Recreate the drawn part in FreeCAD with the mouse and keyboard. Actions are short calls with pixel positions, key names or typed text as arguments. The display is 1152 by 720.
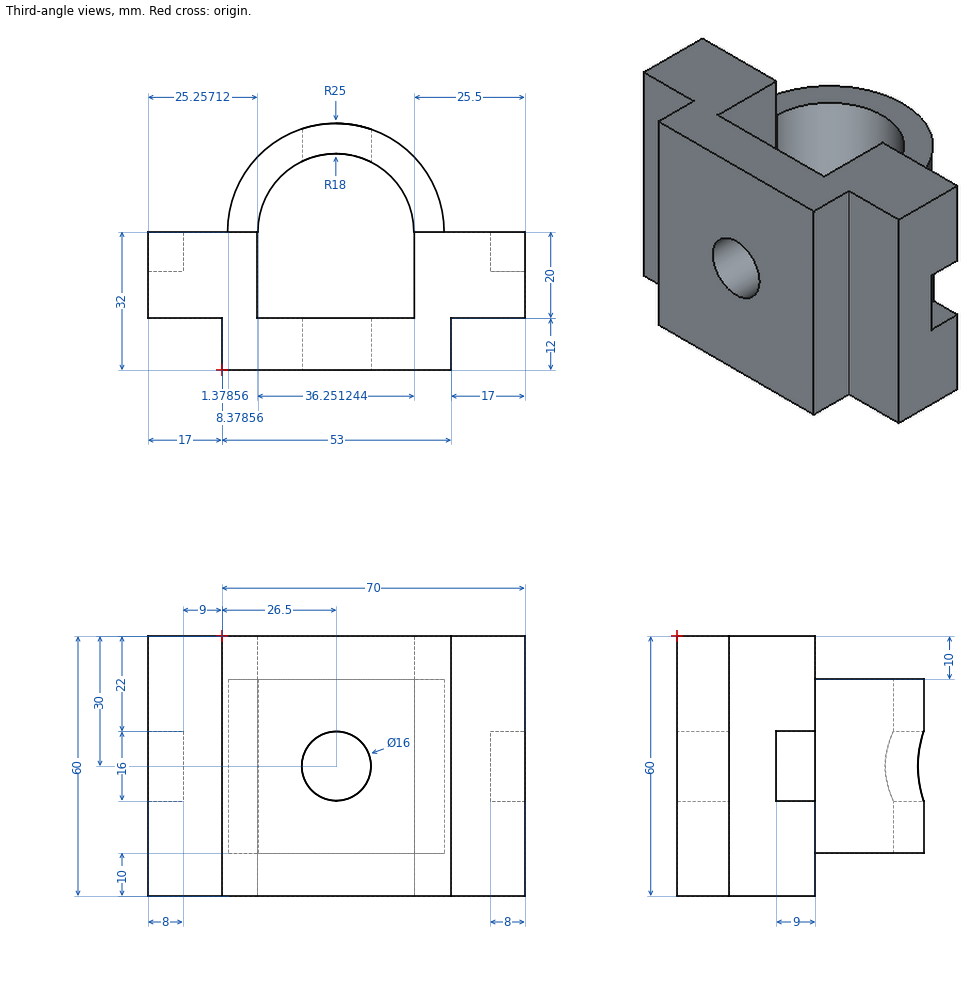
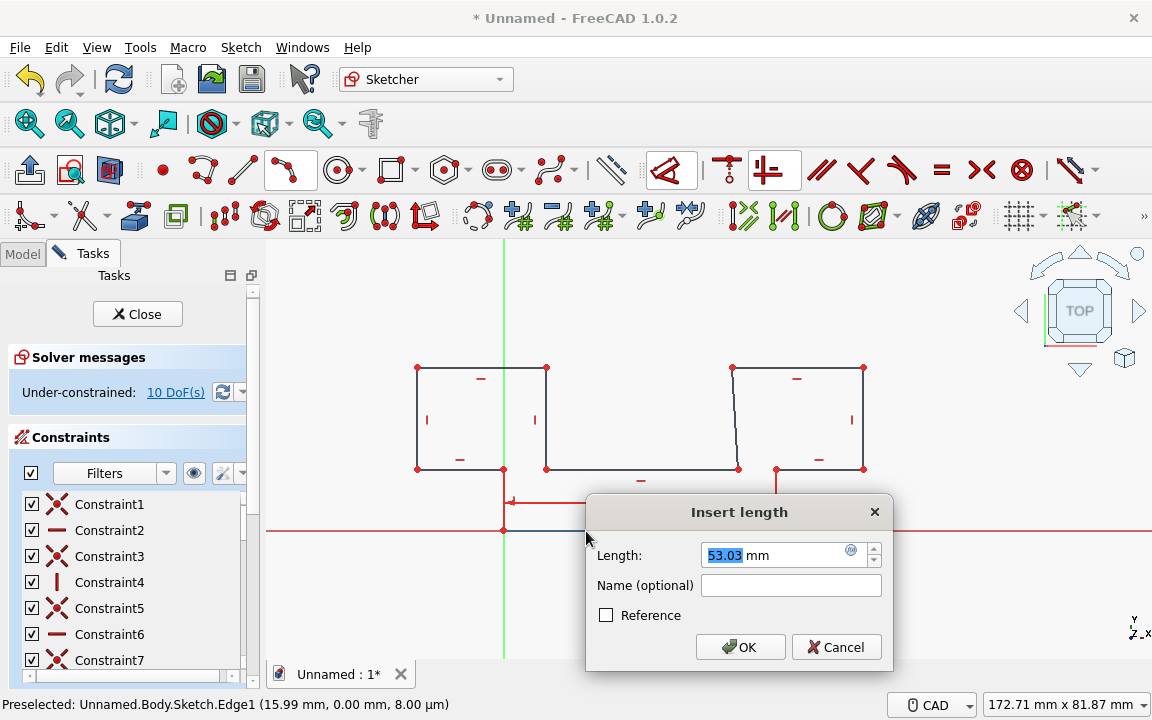
text(53)
key(Return)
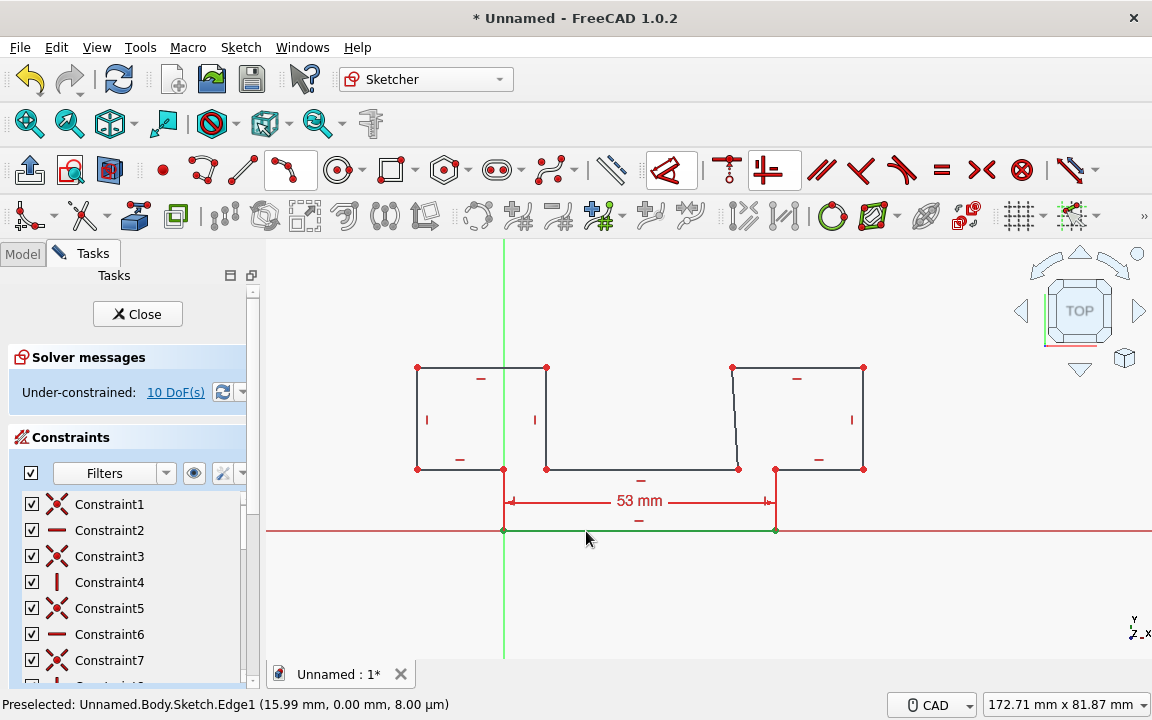
click(776, 513)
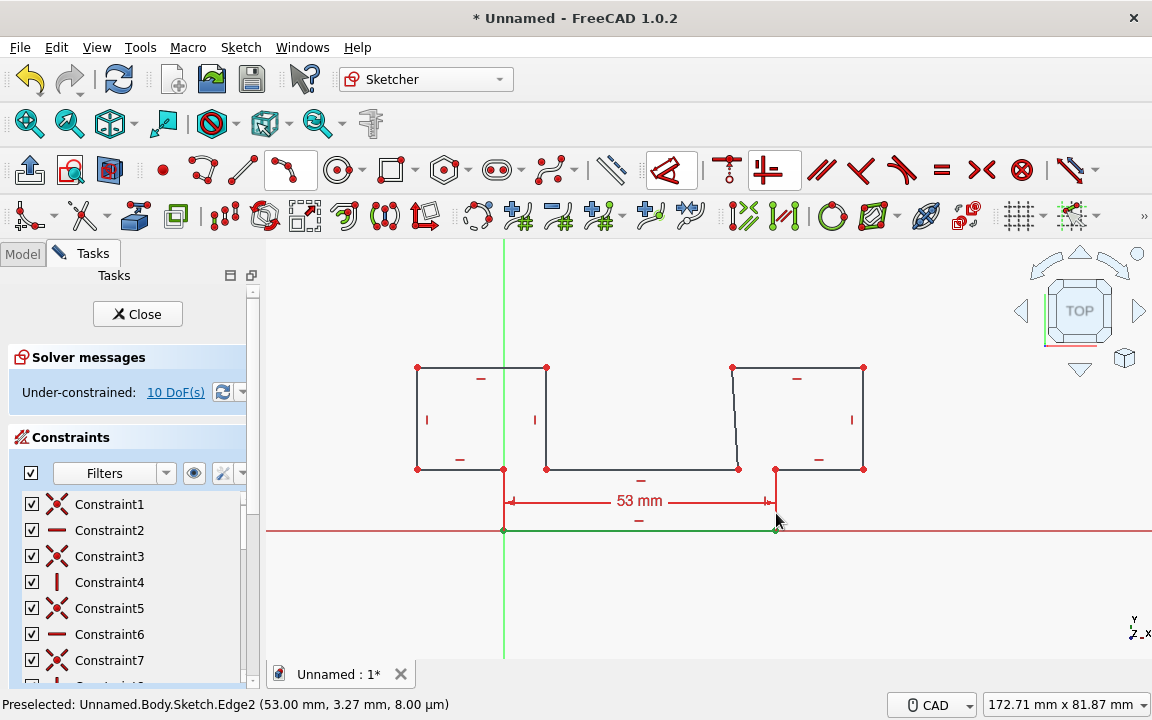
key(i)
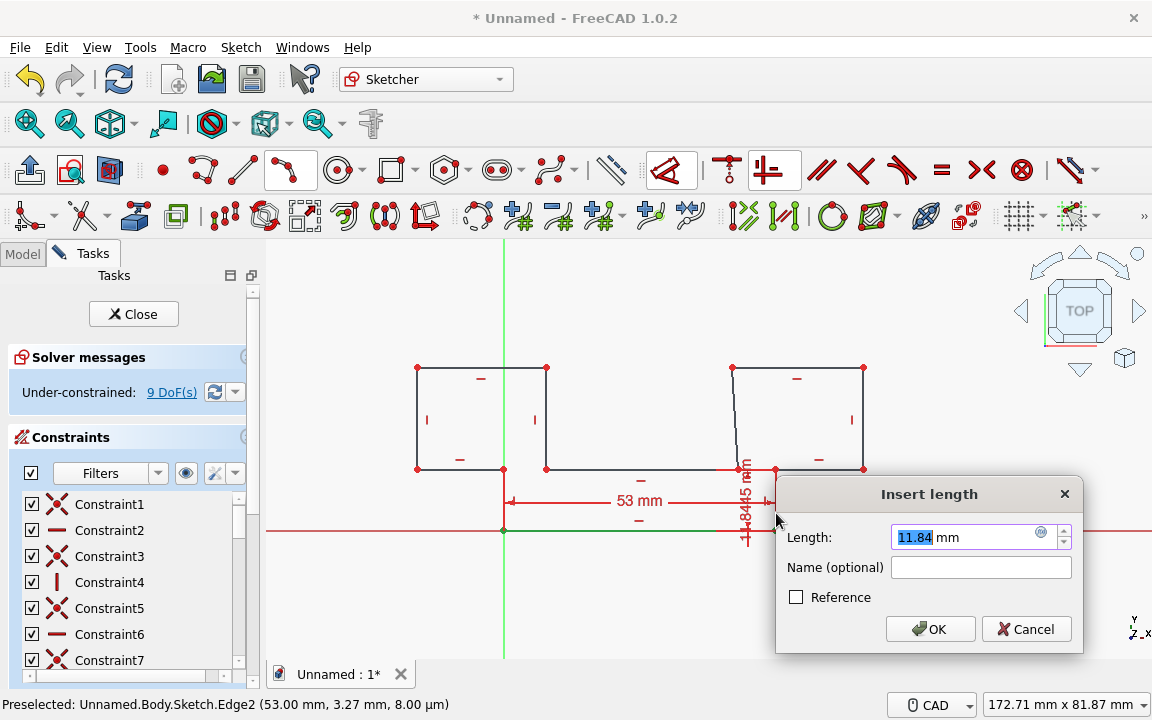
text(12)
key(Return)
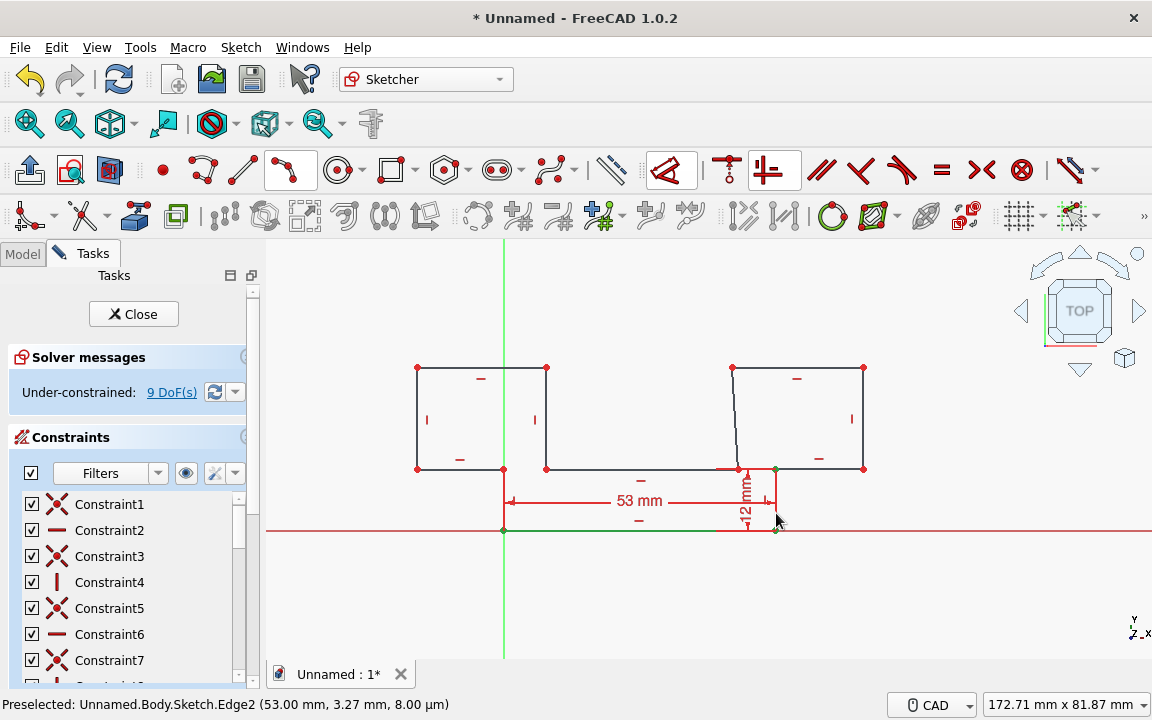
click(802, 469)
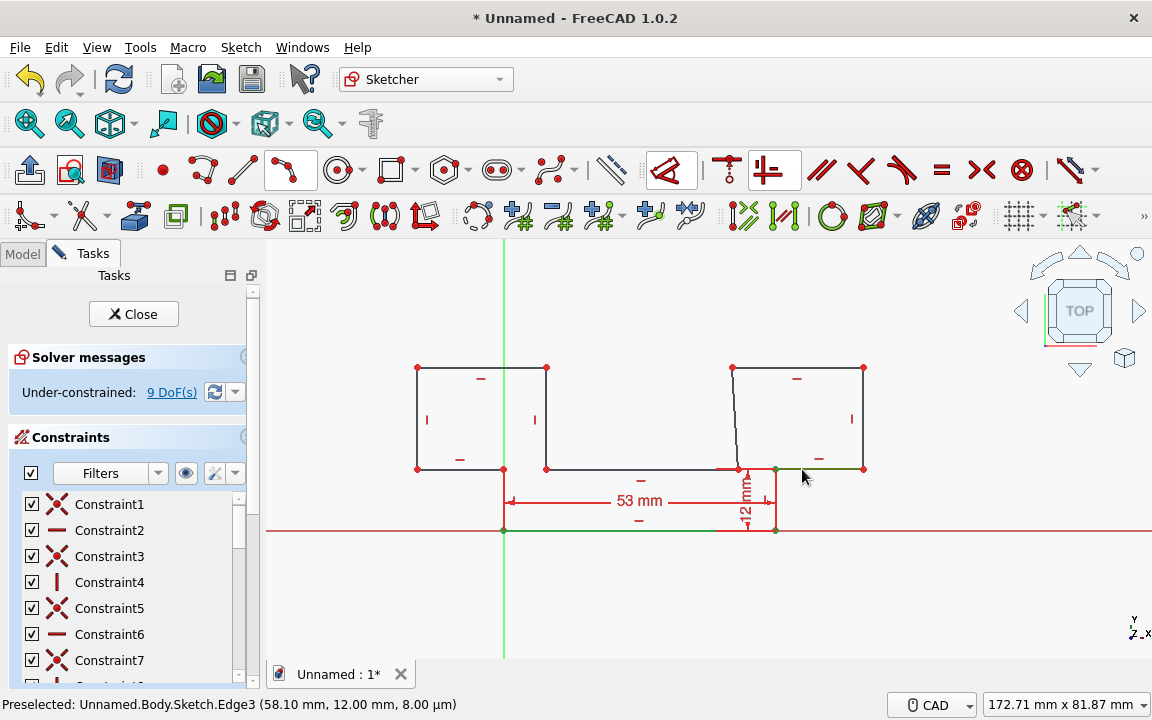
key(l)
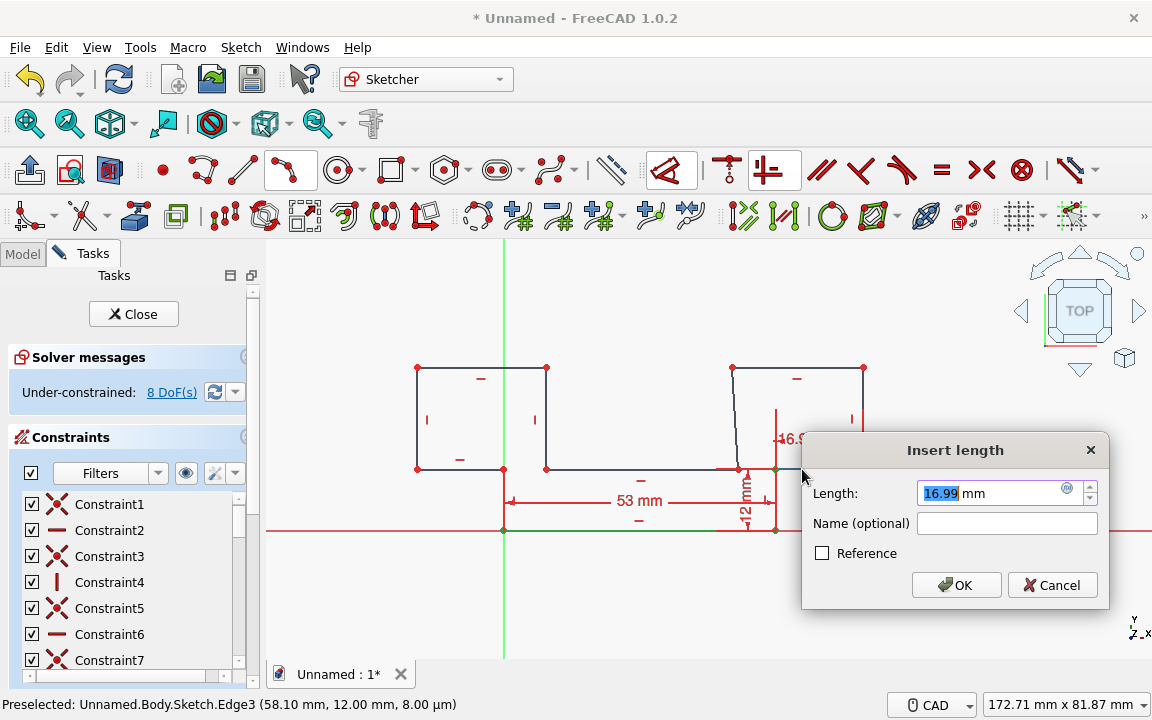
text(17)
key(Return)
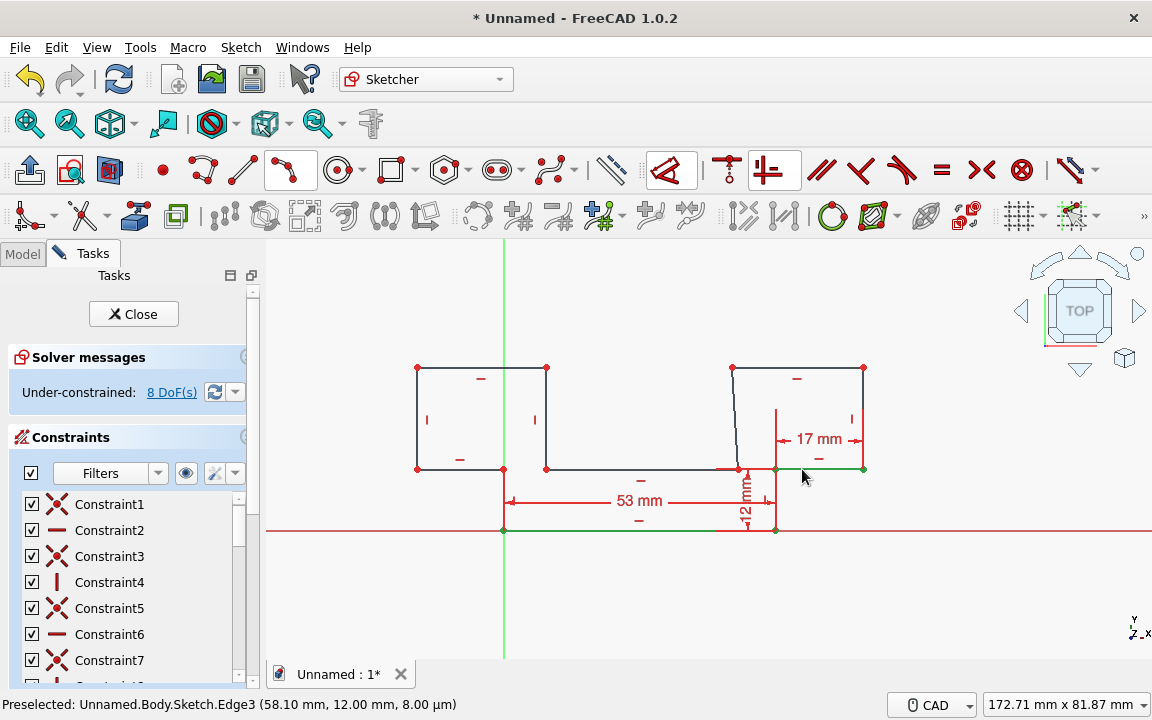
click(863, 439)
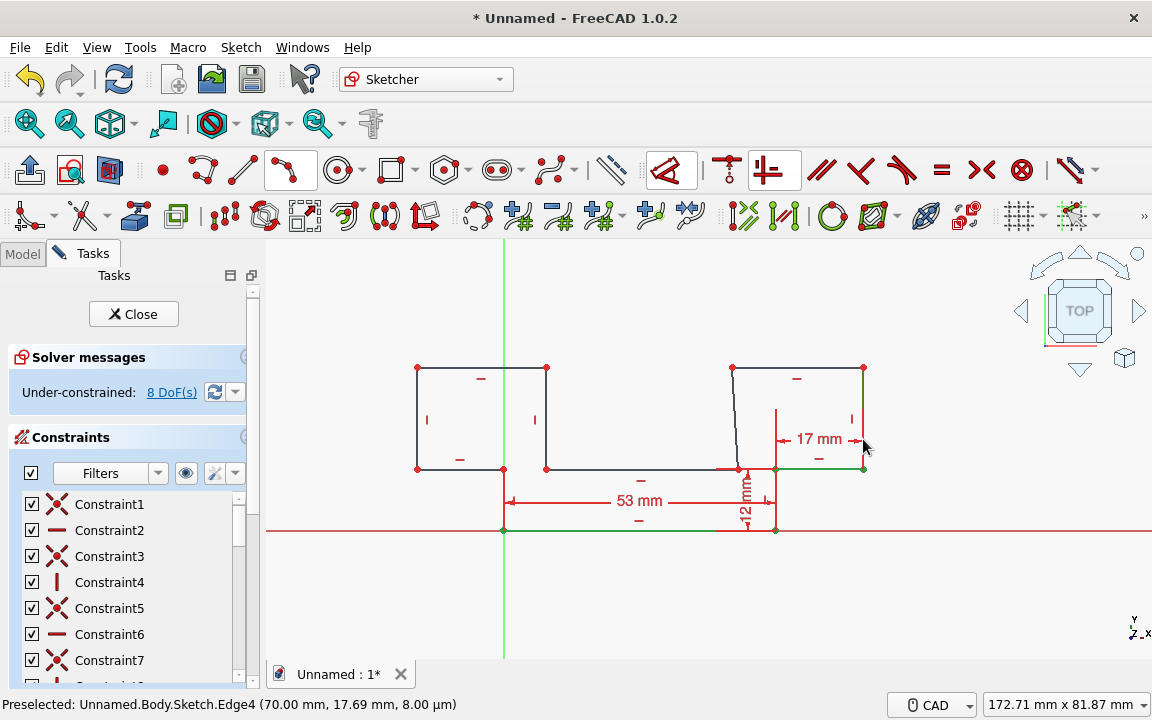
click(692, 170)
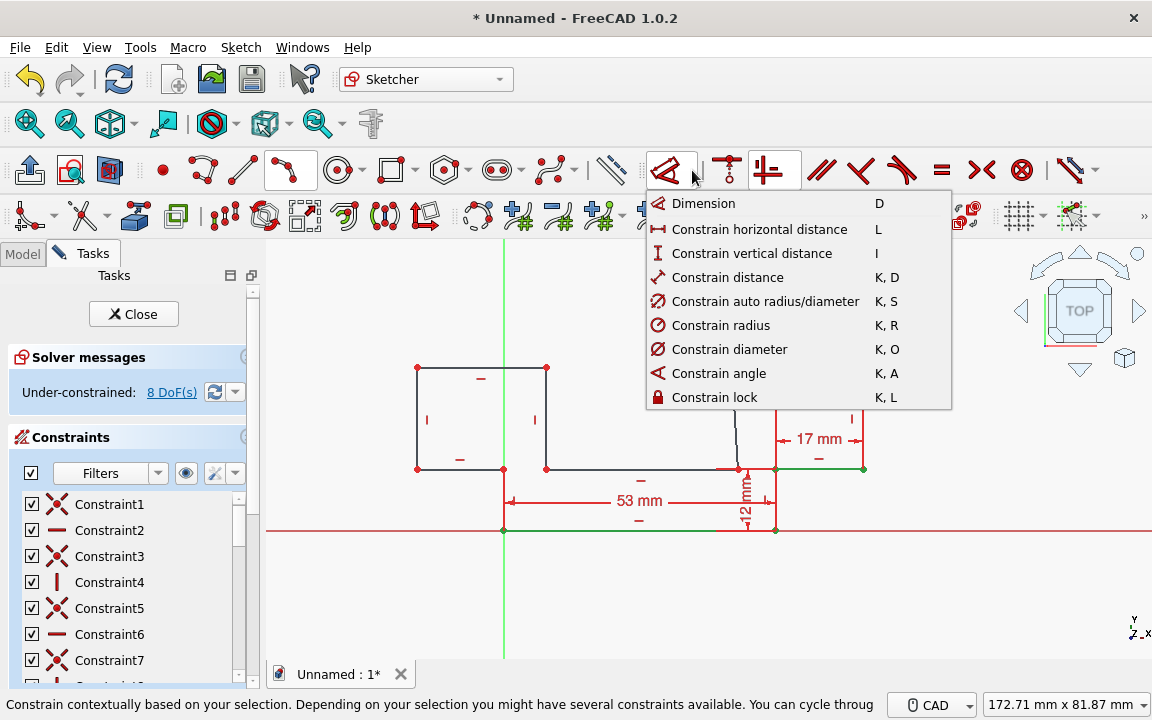
click(799, 253)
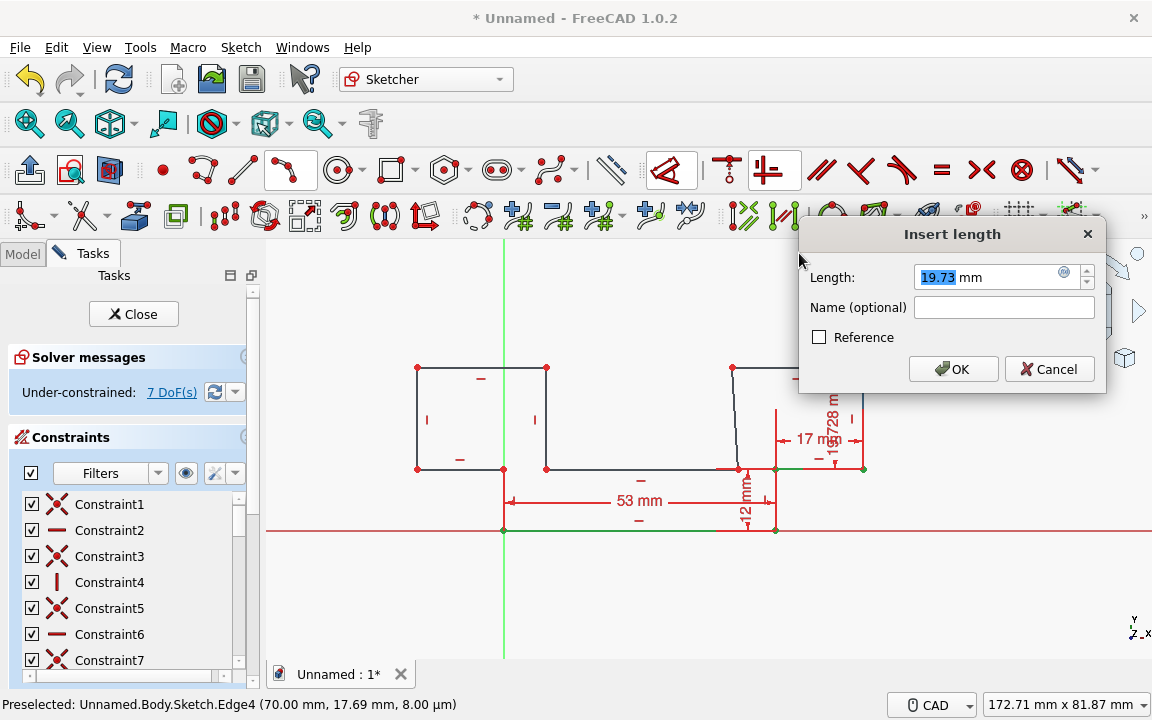
text(20)
key(Return)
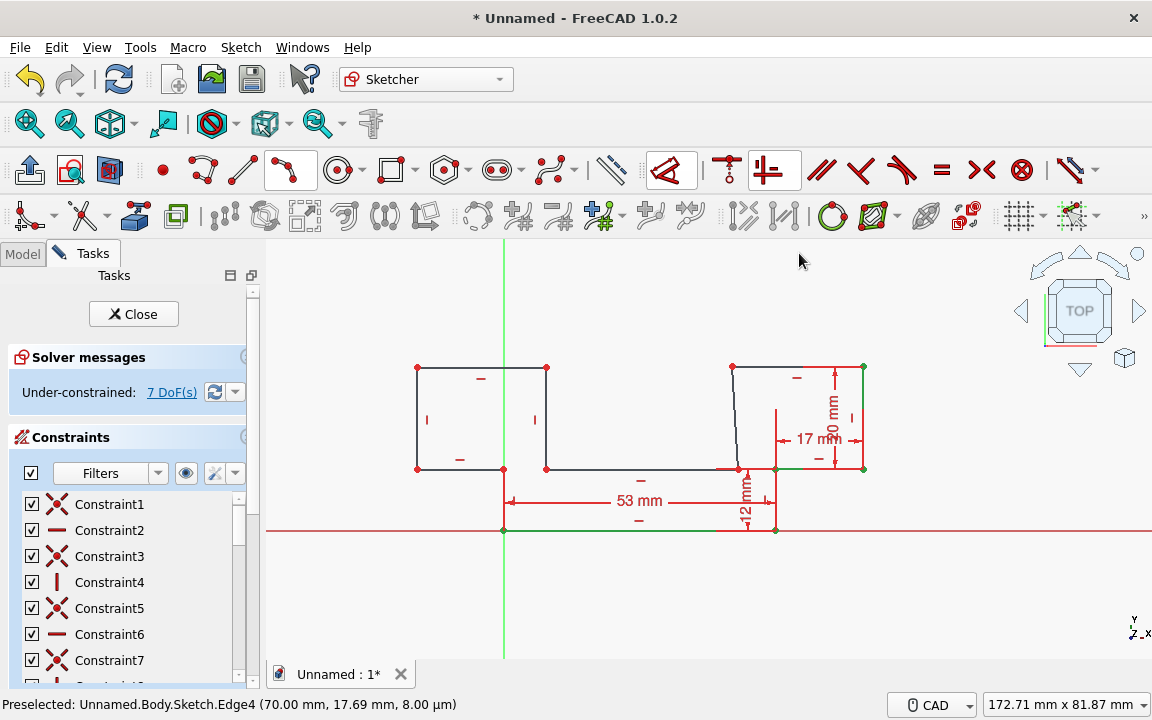
click(546, 439)